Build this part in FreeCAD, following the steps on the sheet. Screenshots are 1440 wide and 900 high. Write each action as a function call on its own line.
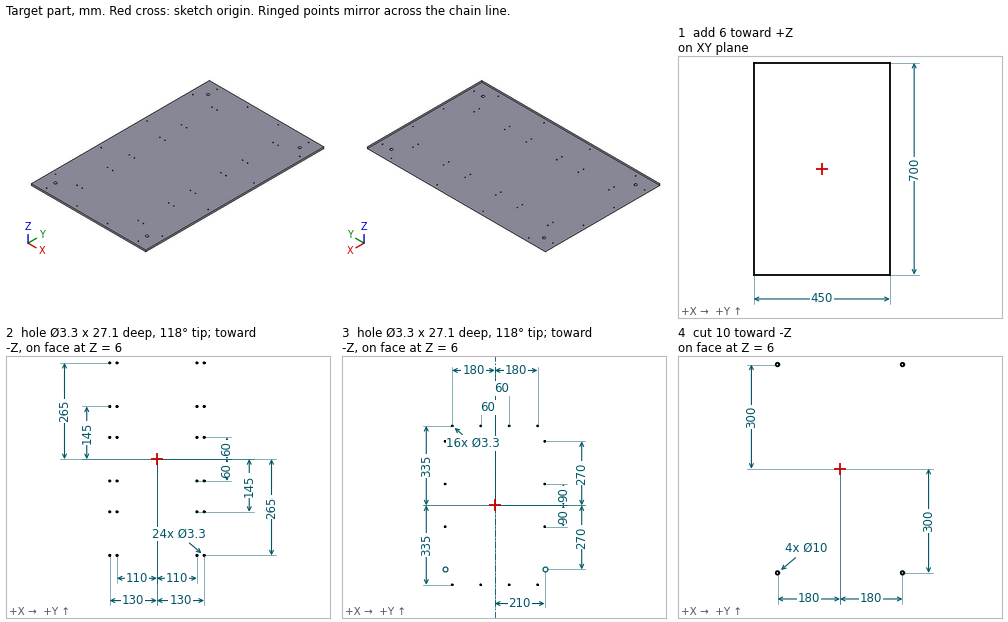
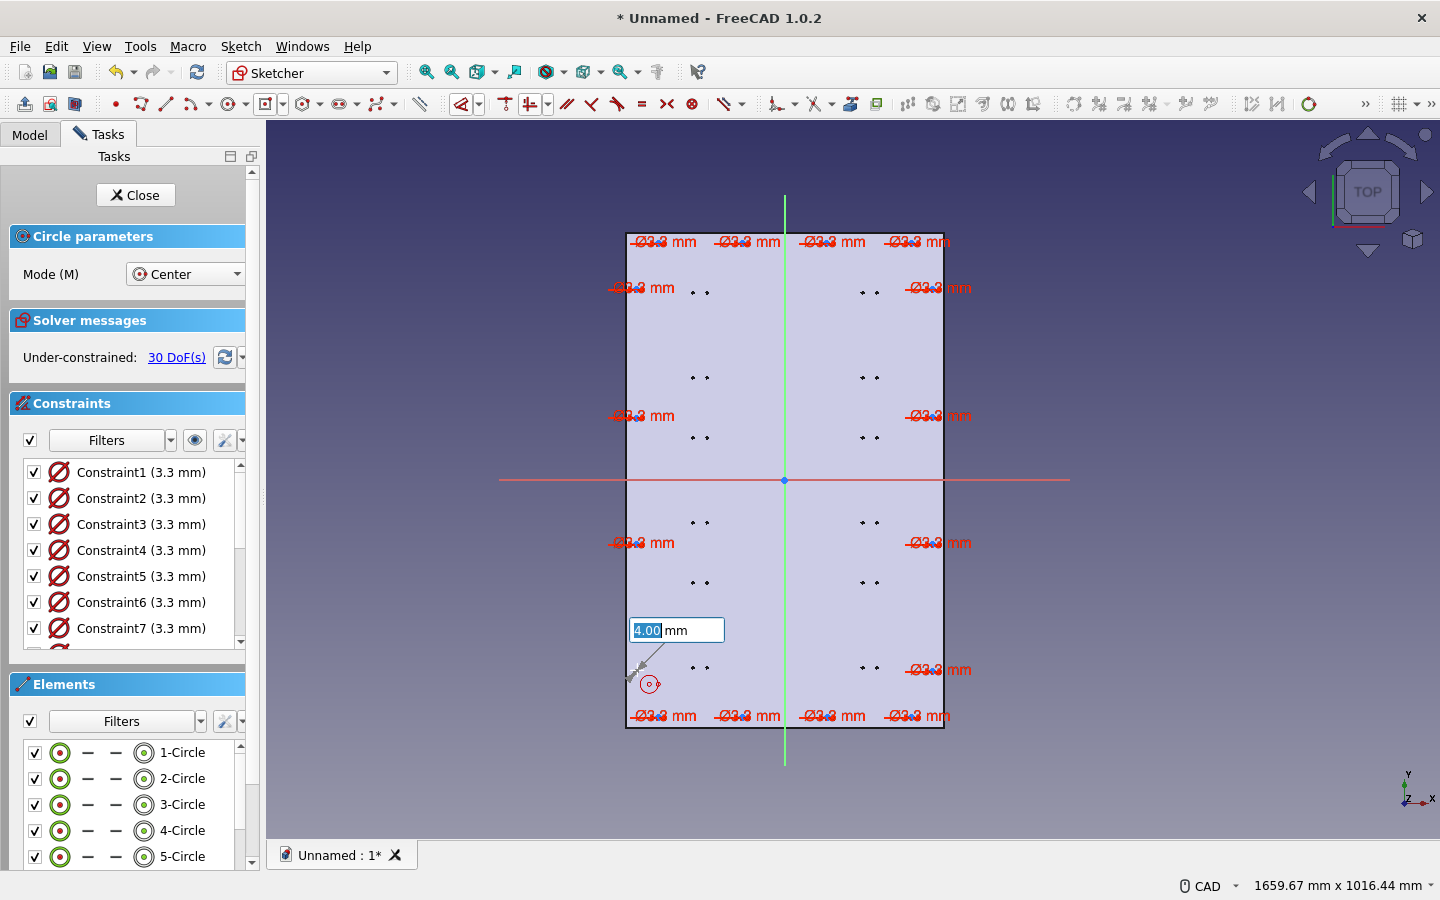
text(3.3)
key(Return)
key(Escape)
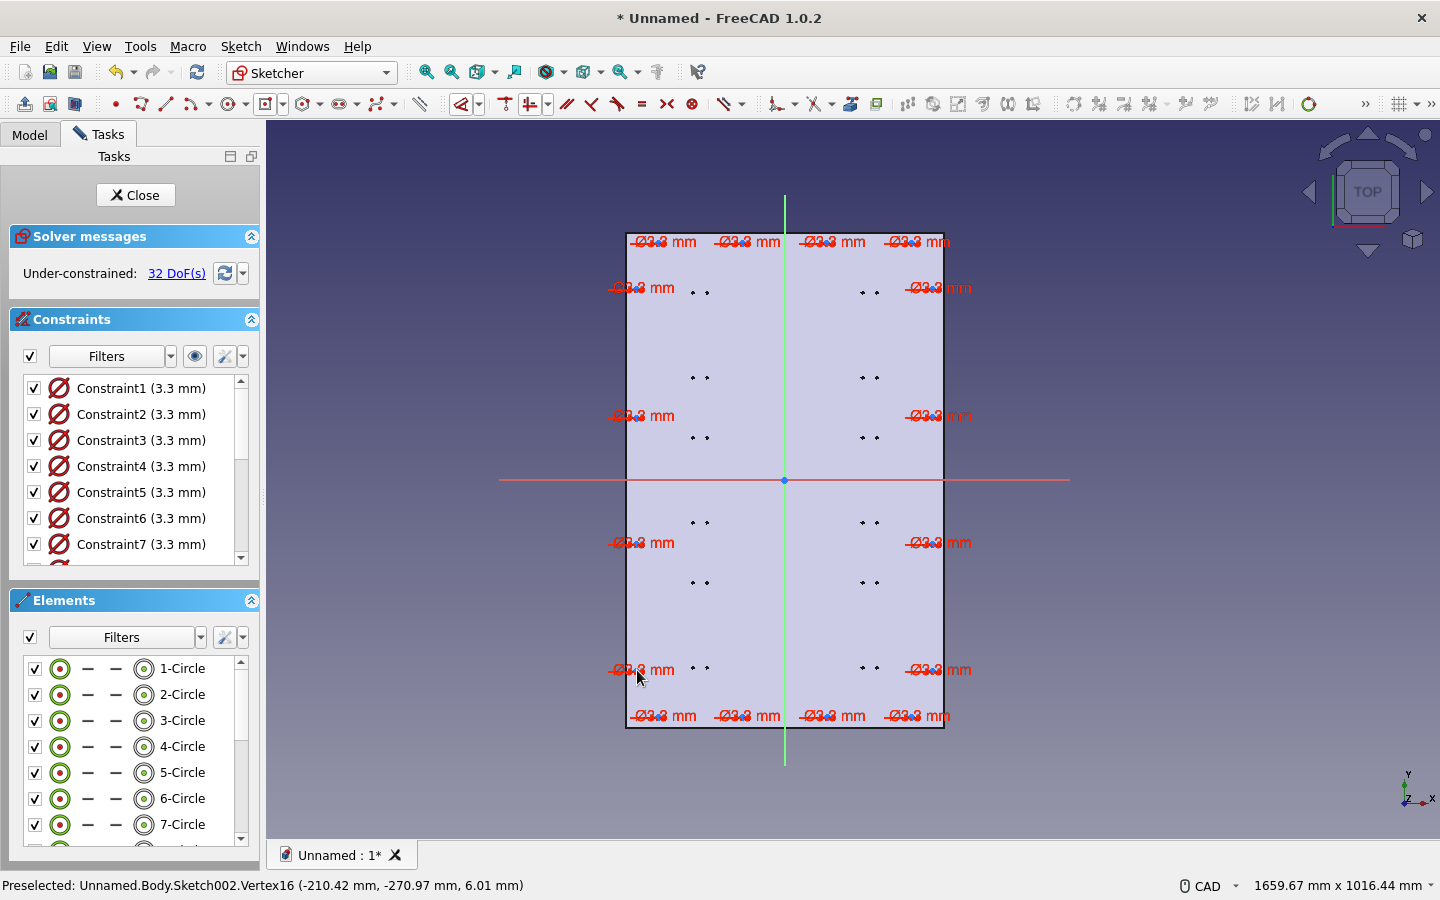
click(658, 244)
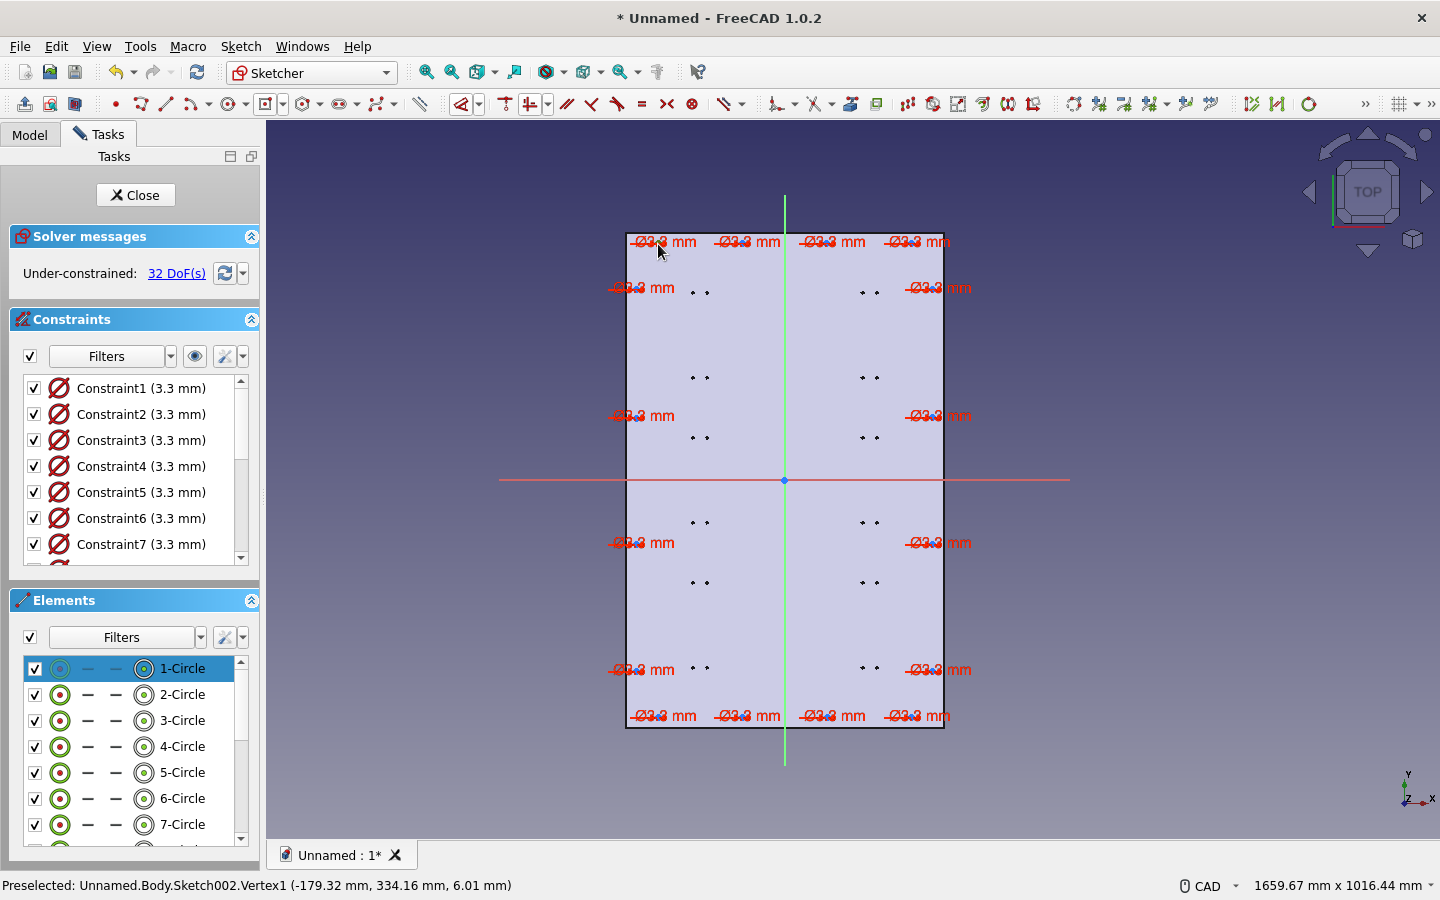
click(742, 244)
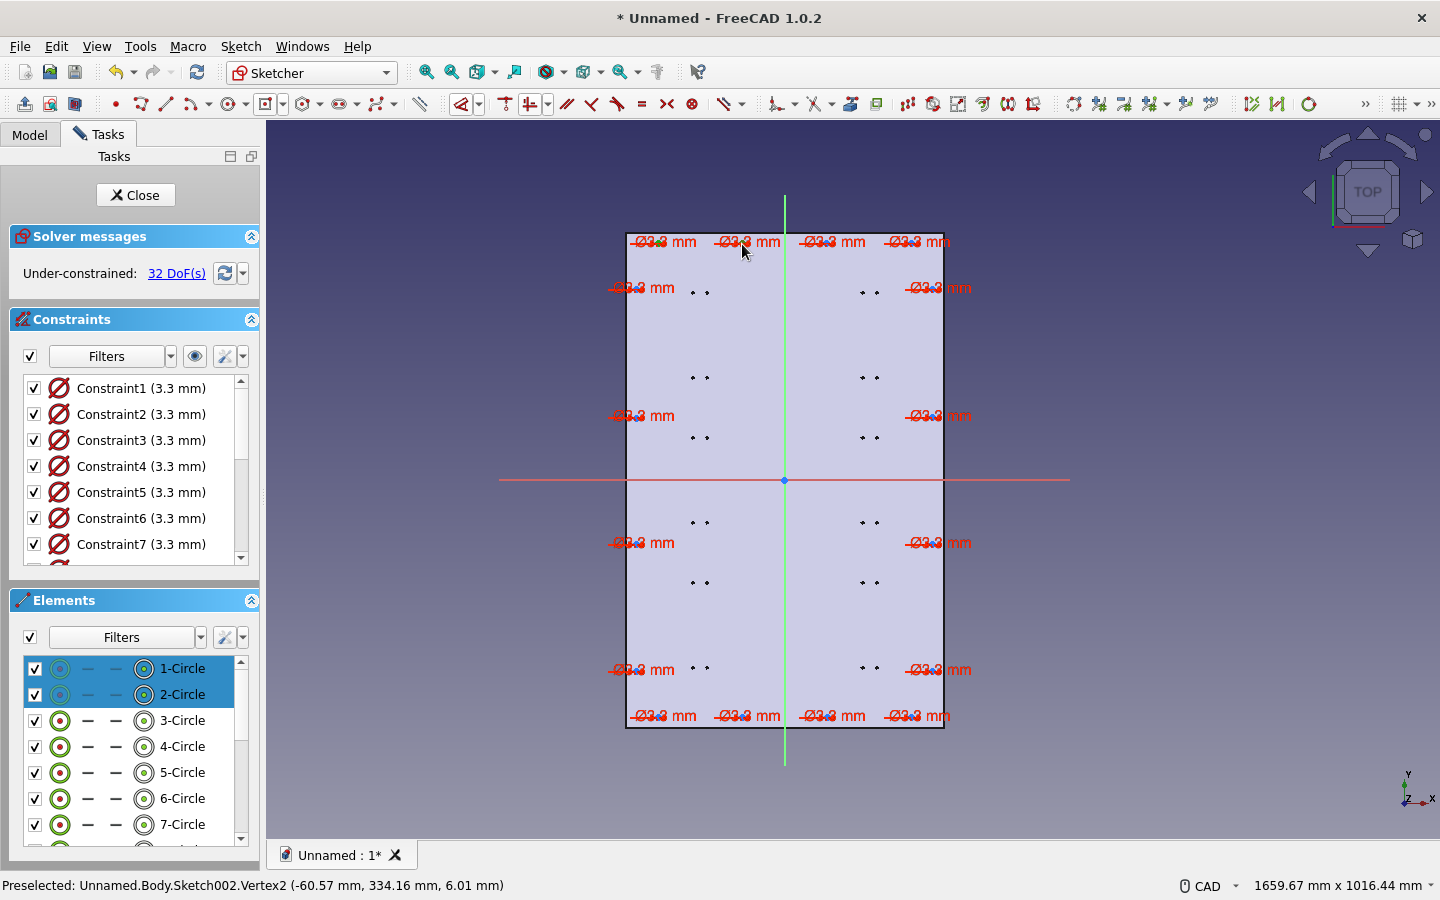
click(548, 104)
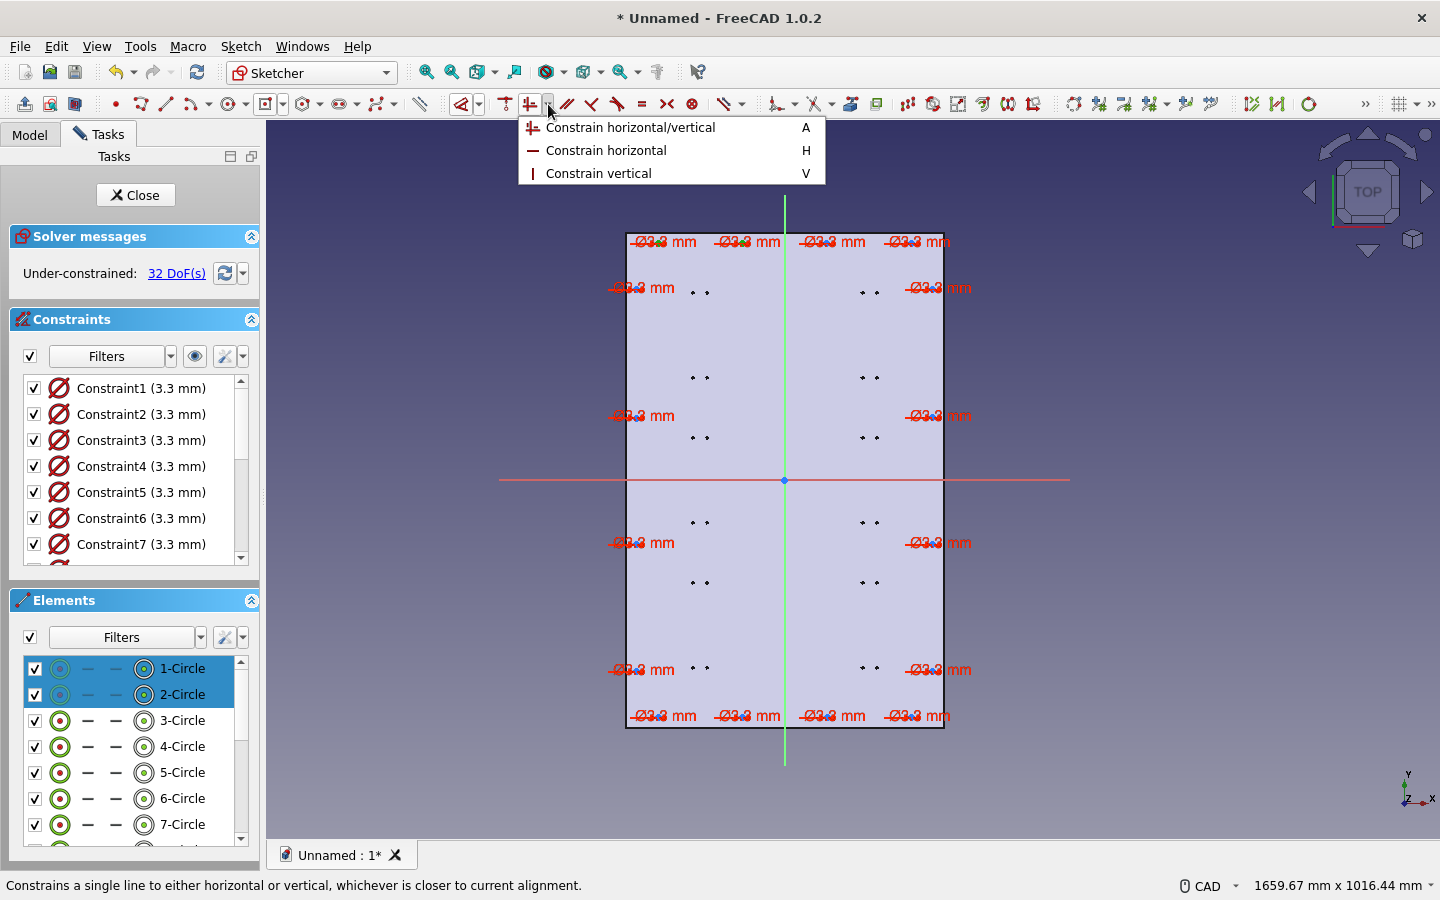
click(672, 150)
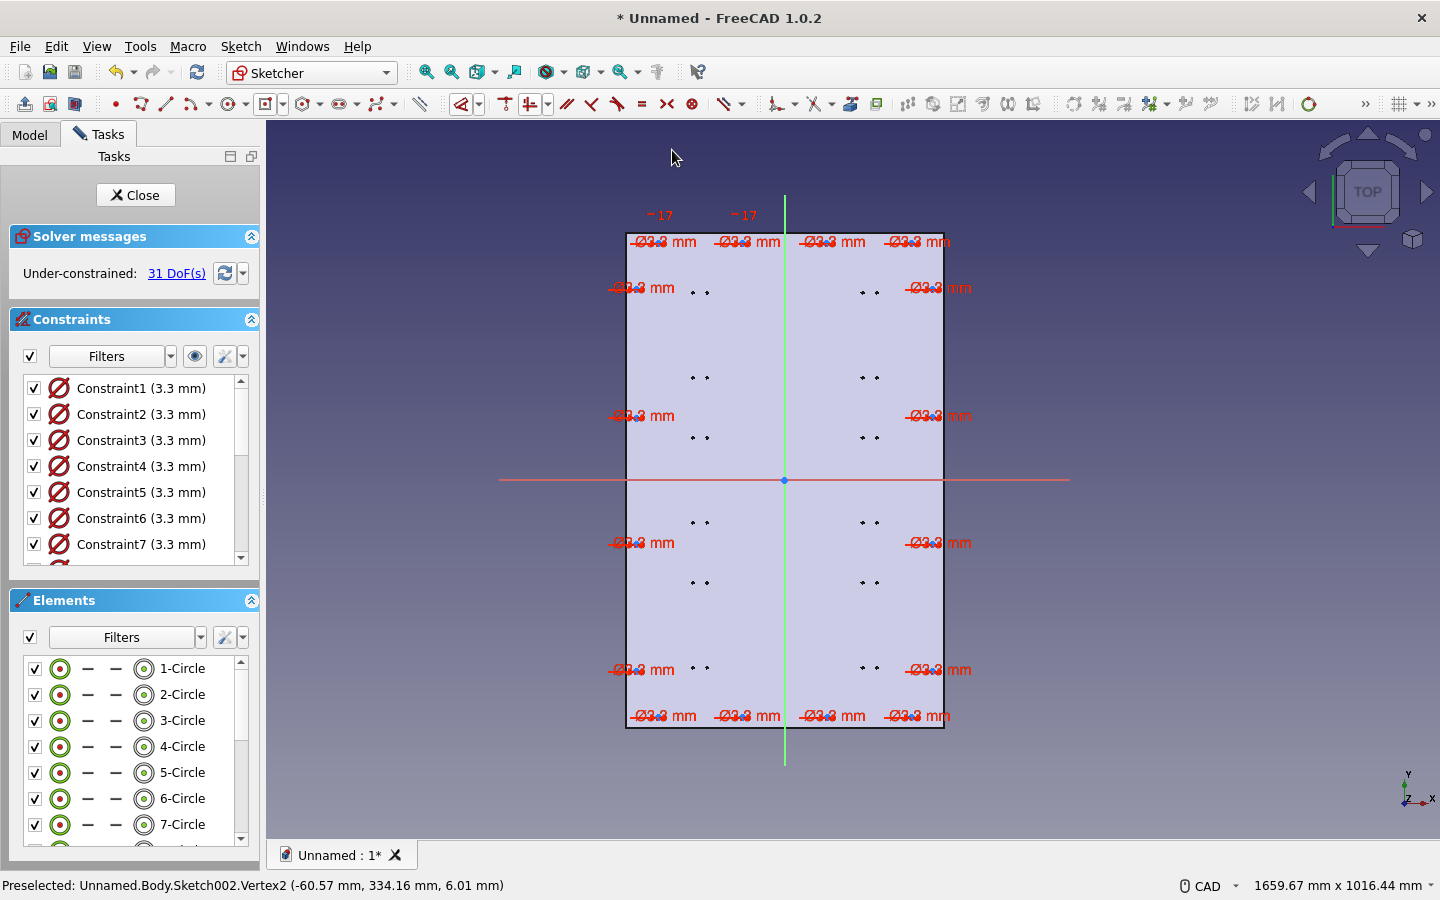
click(742, 244)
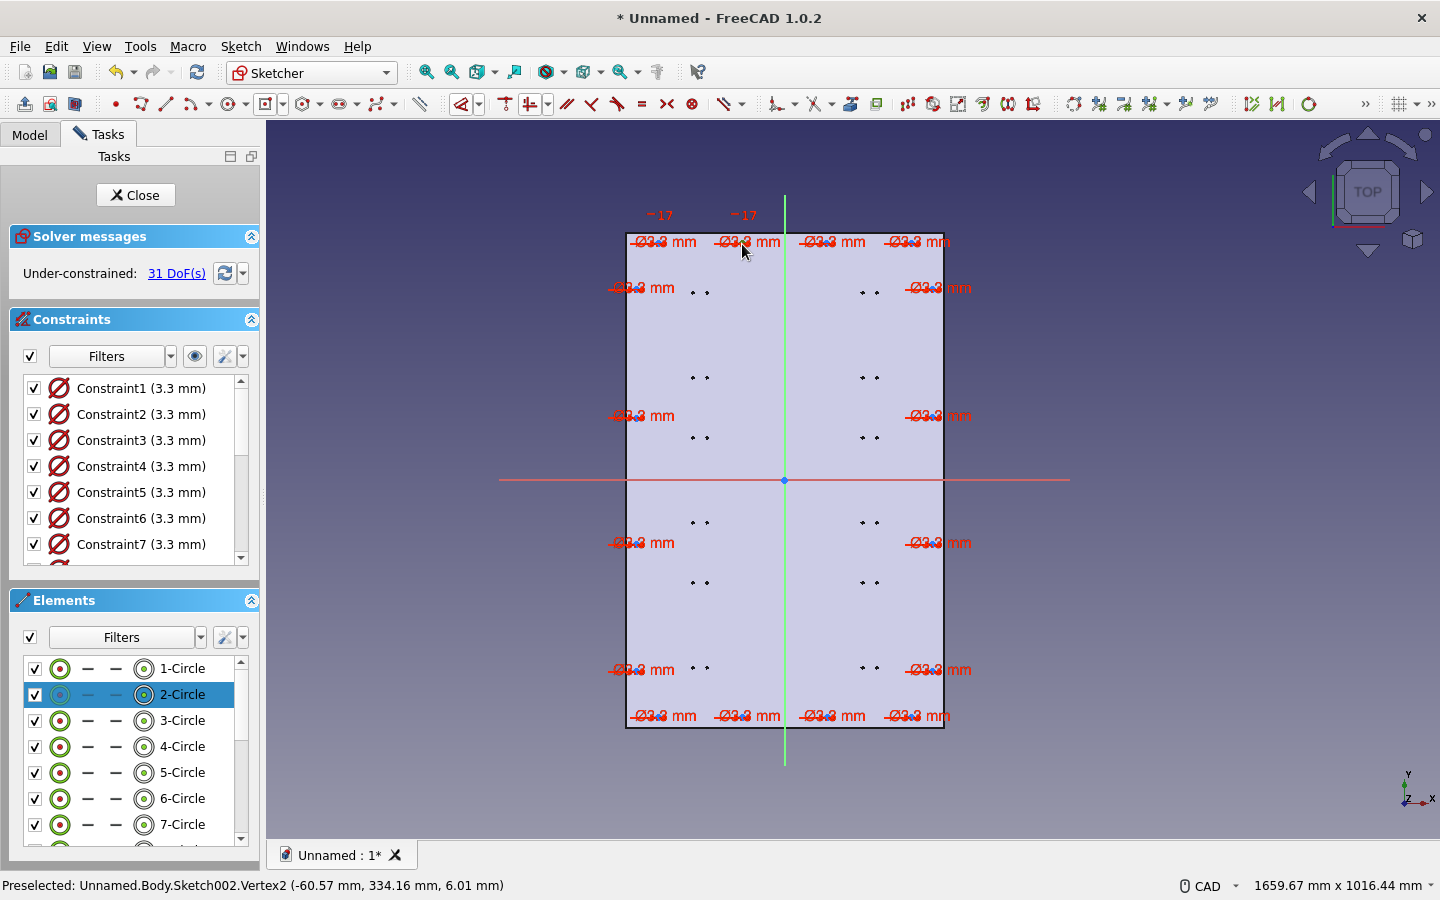
click(827, 244)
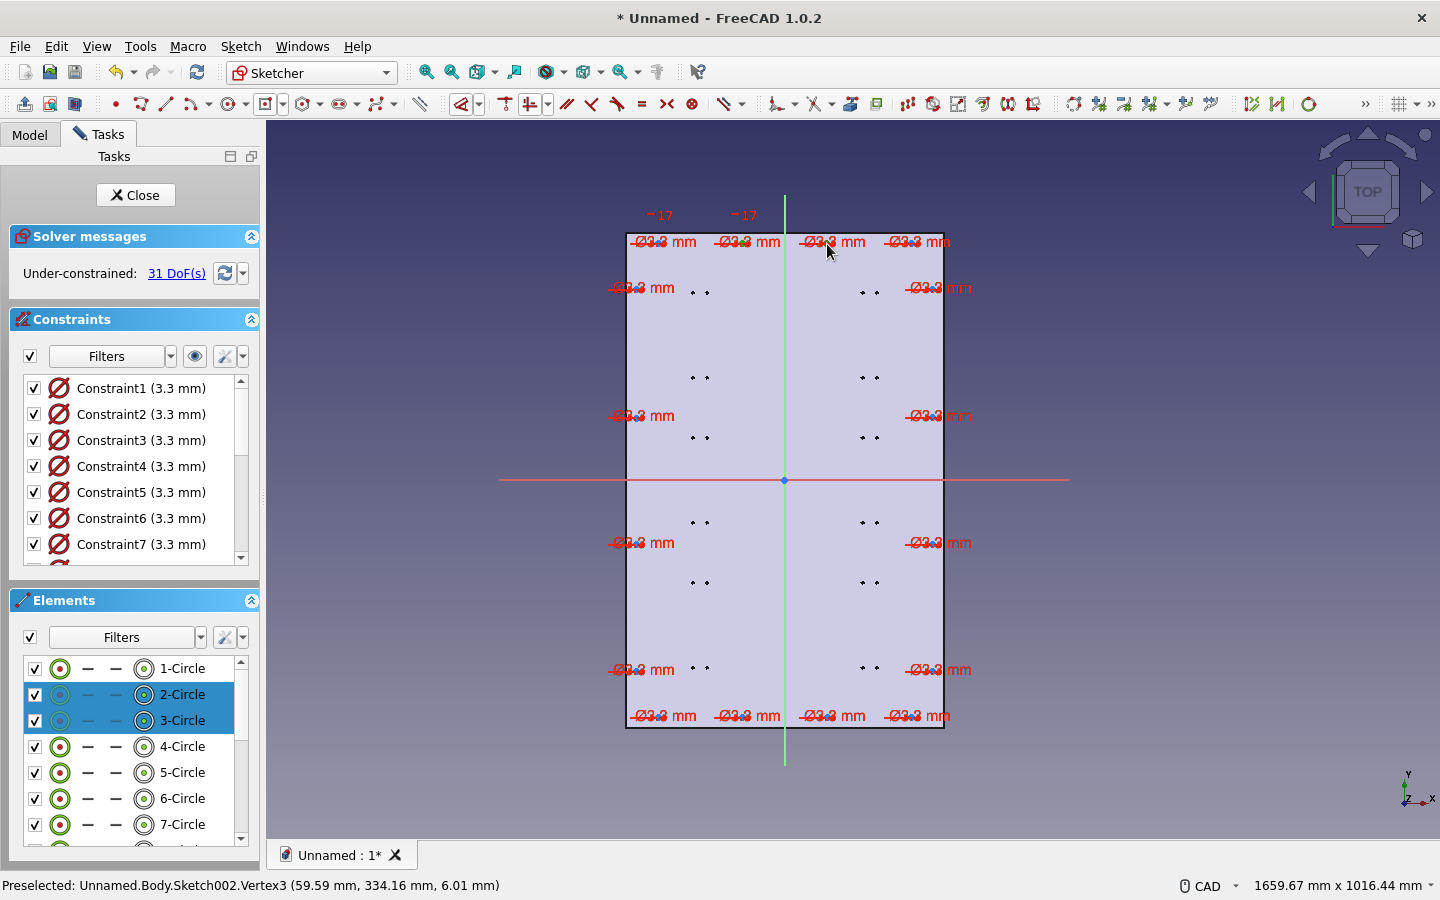
click(548, 104)